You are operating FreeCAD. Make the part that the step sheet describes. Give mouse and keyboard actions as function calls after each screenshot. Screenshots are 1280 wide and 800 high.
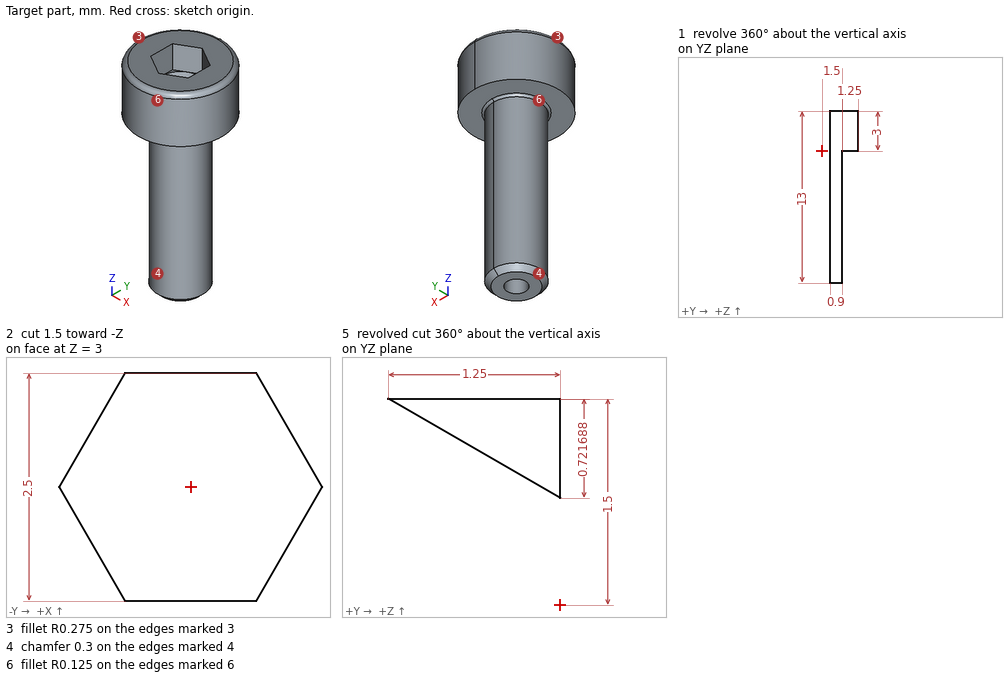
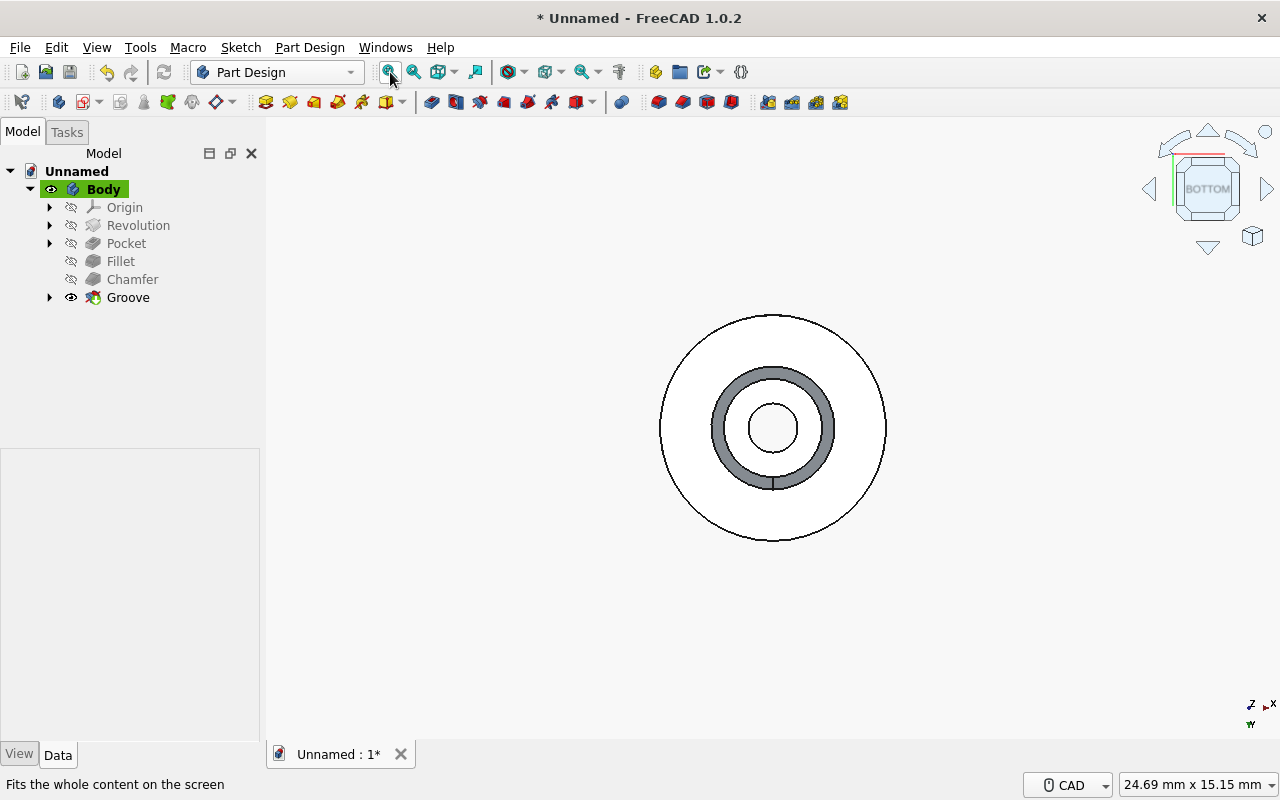
click(390, 72)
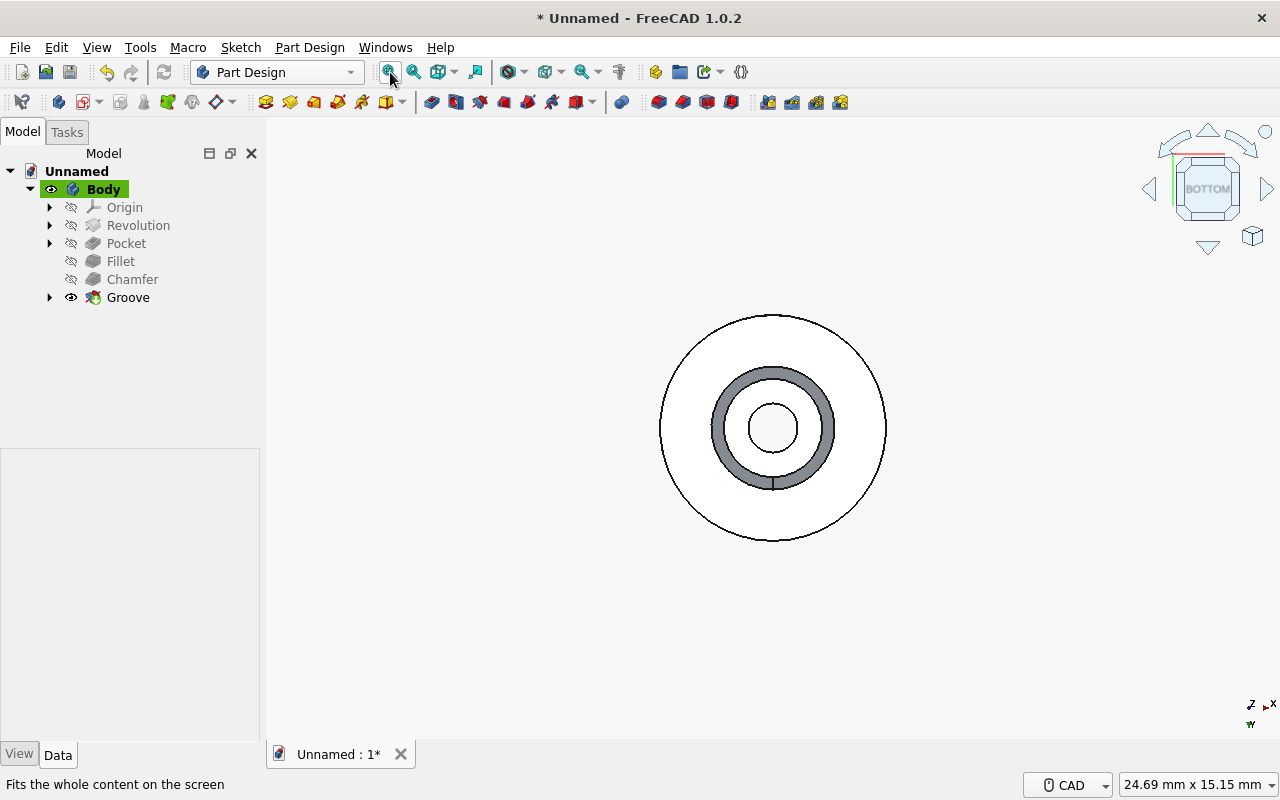
key(4)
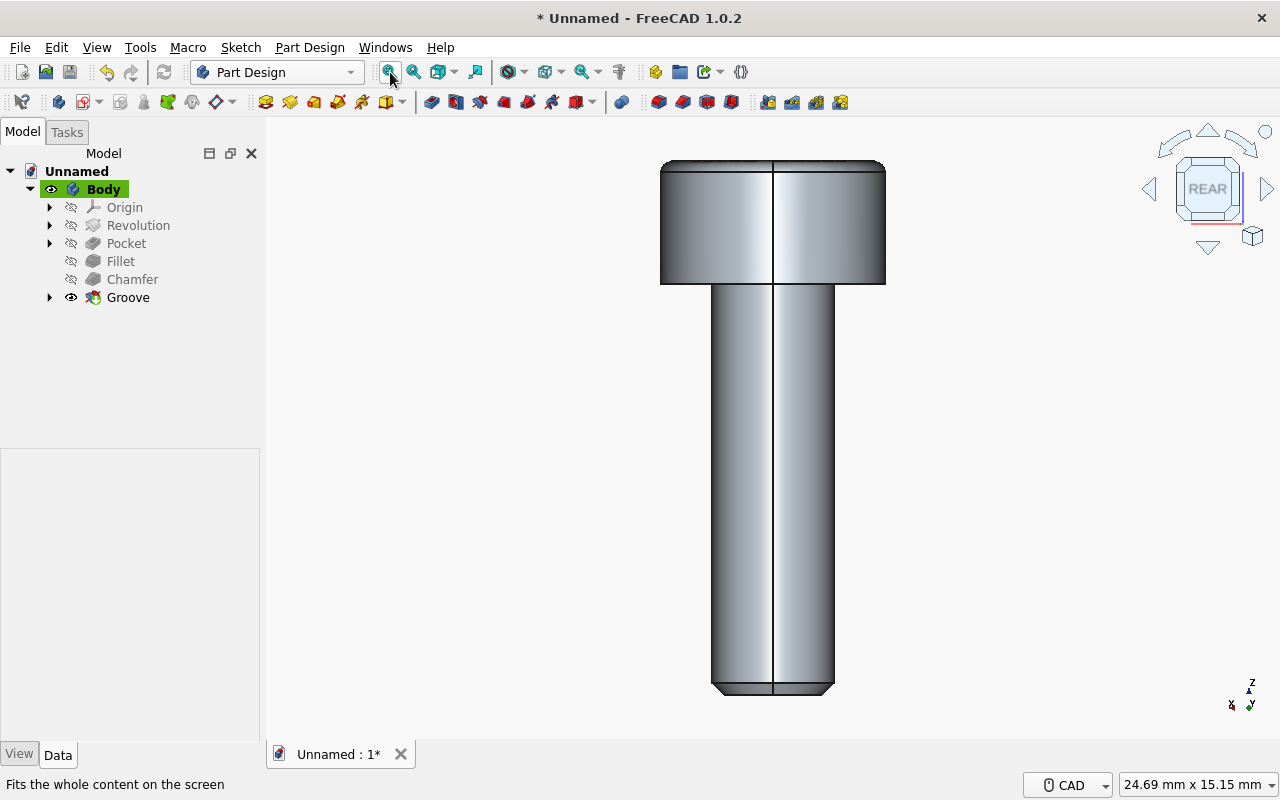
key(6)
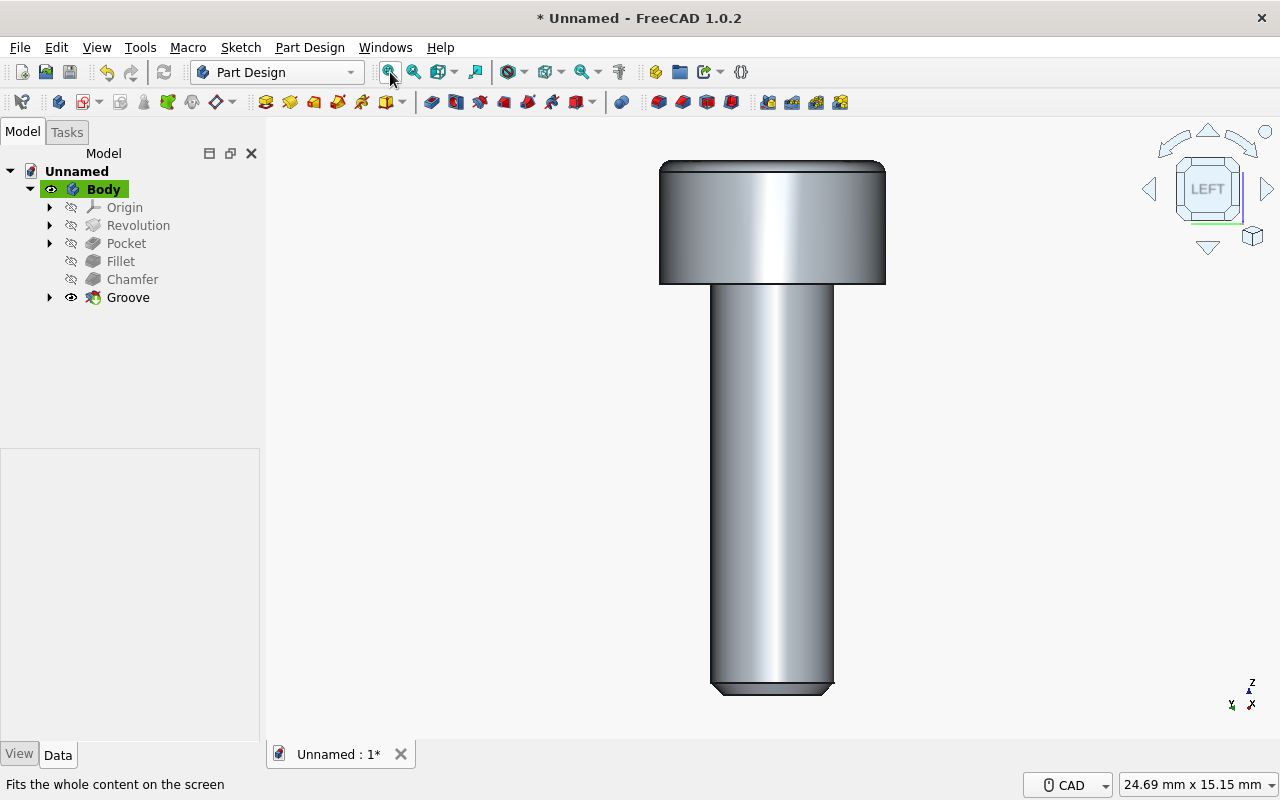
key(v)
key(3)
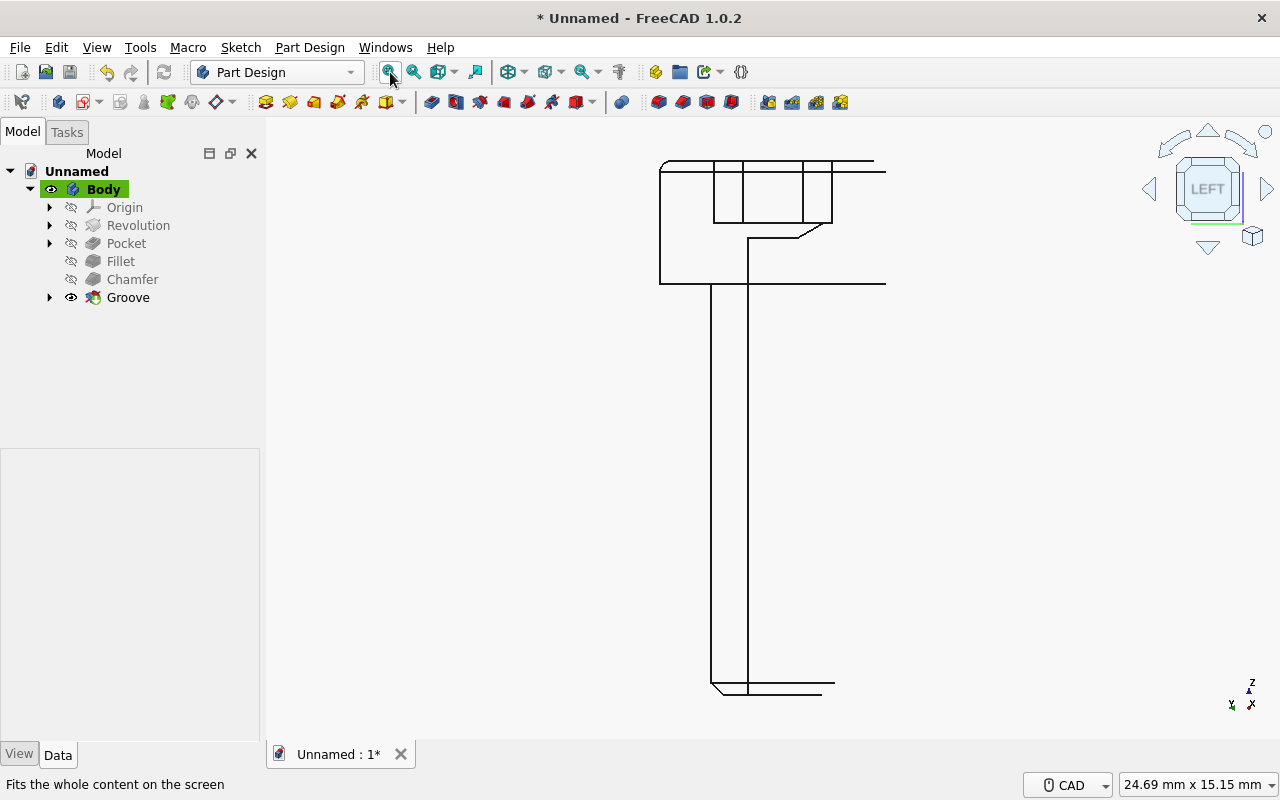
key(0)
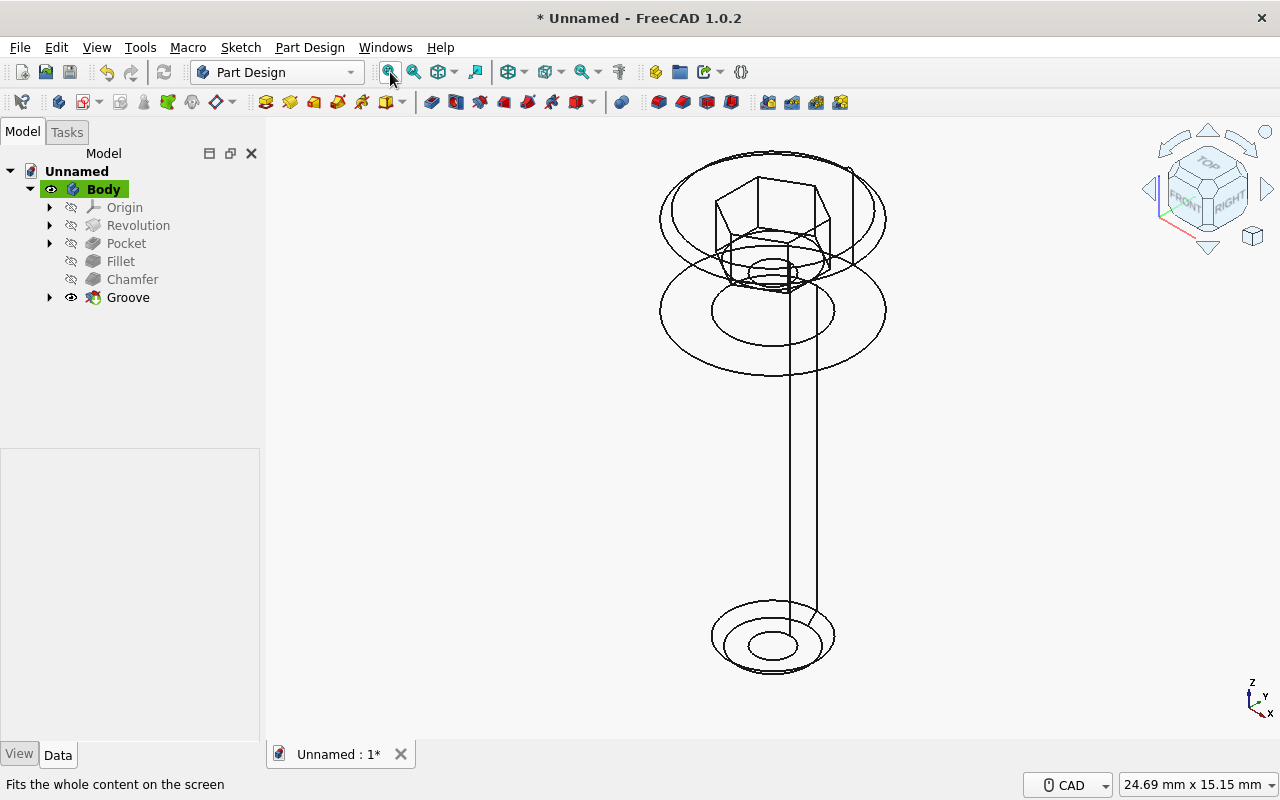
click(729, 335)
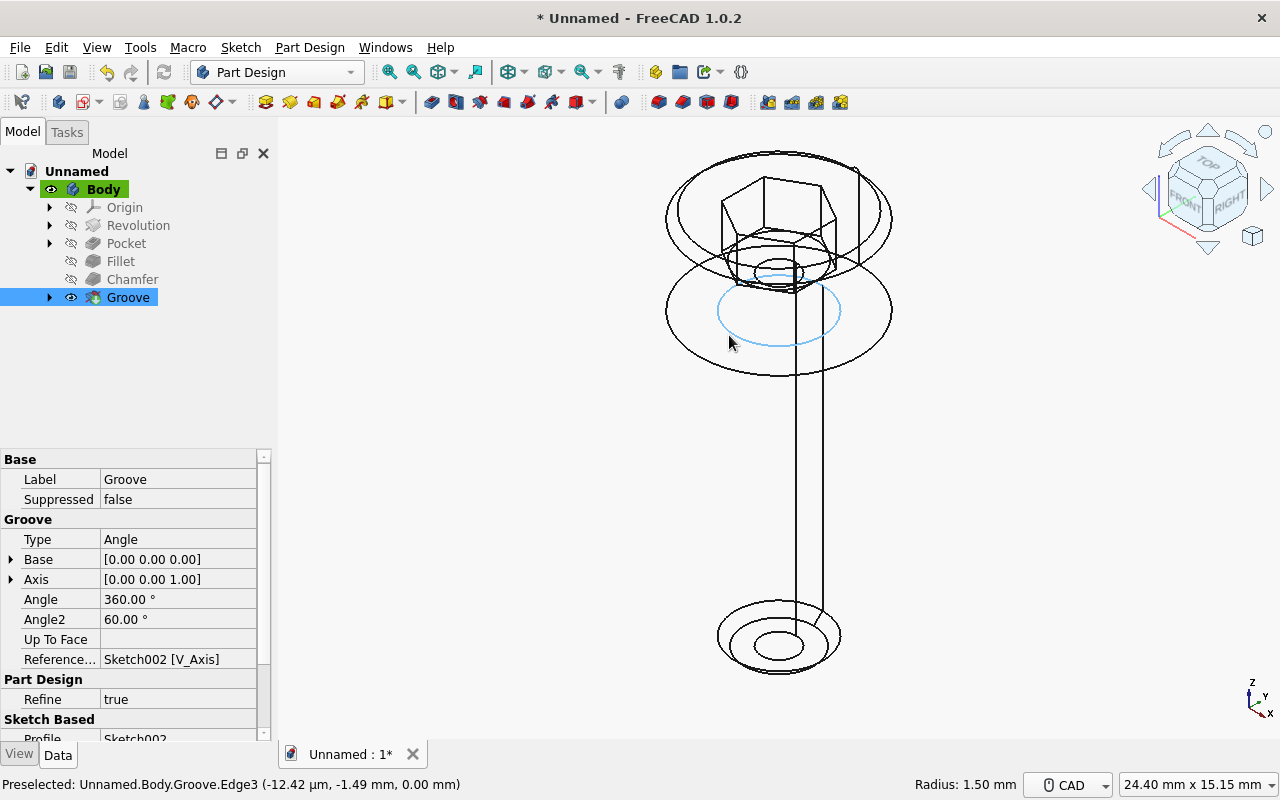
key(v)
key(1)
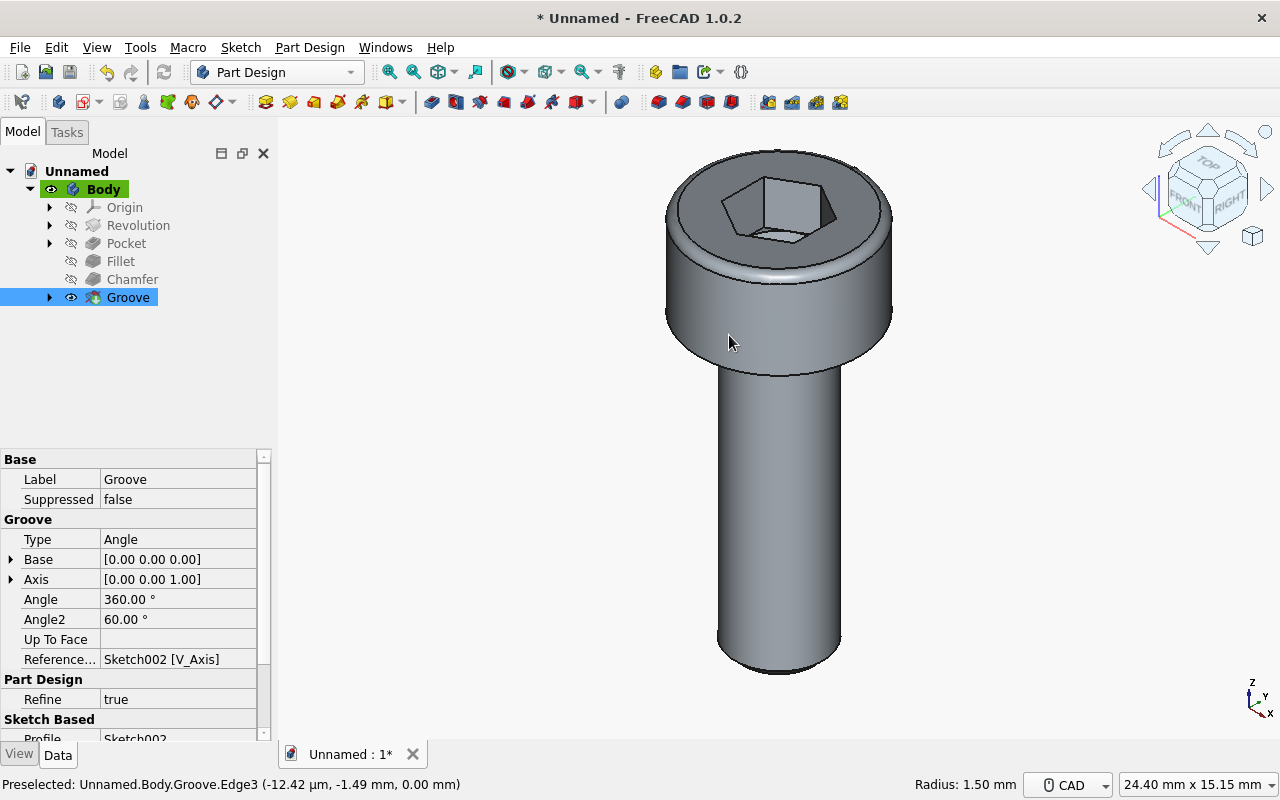
click(660, 102)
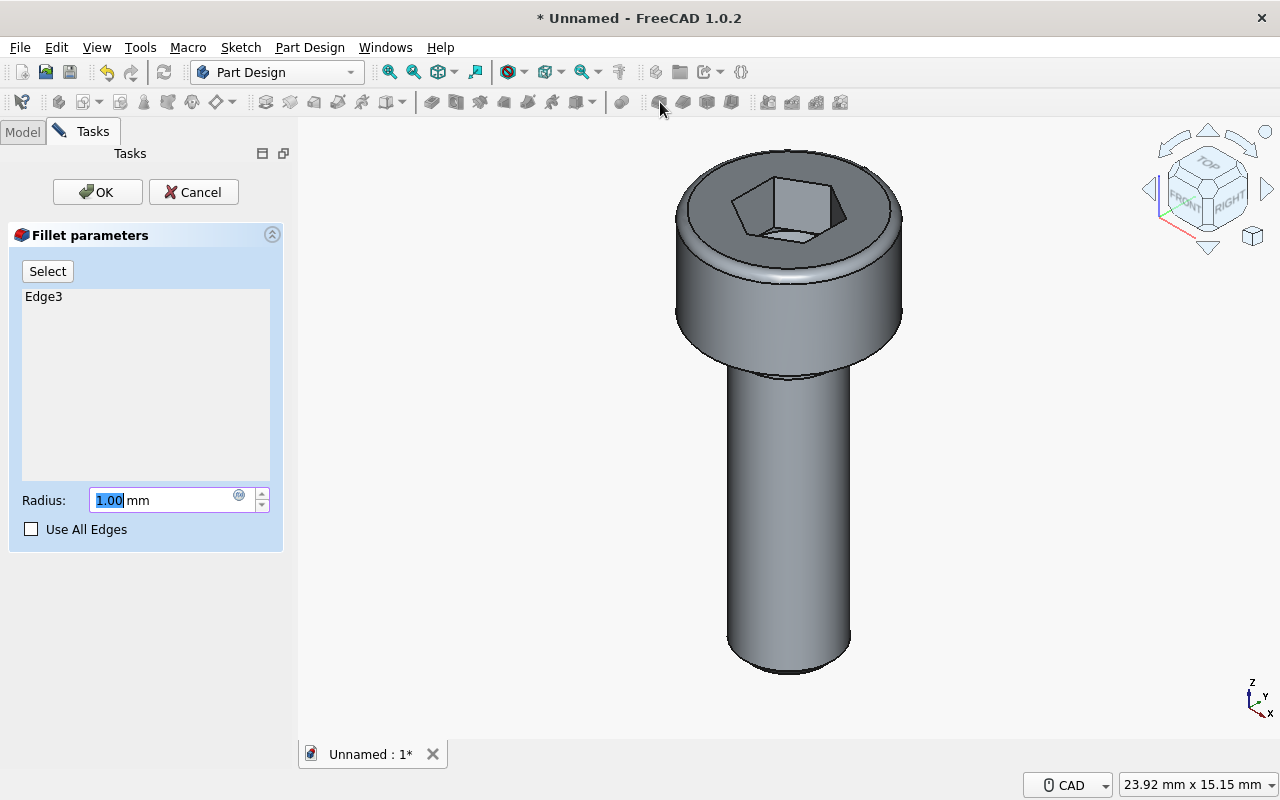
text(0.125)
key(Tab)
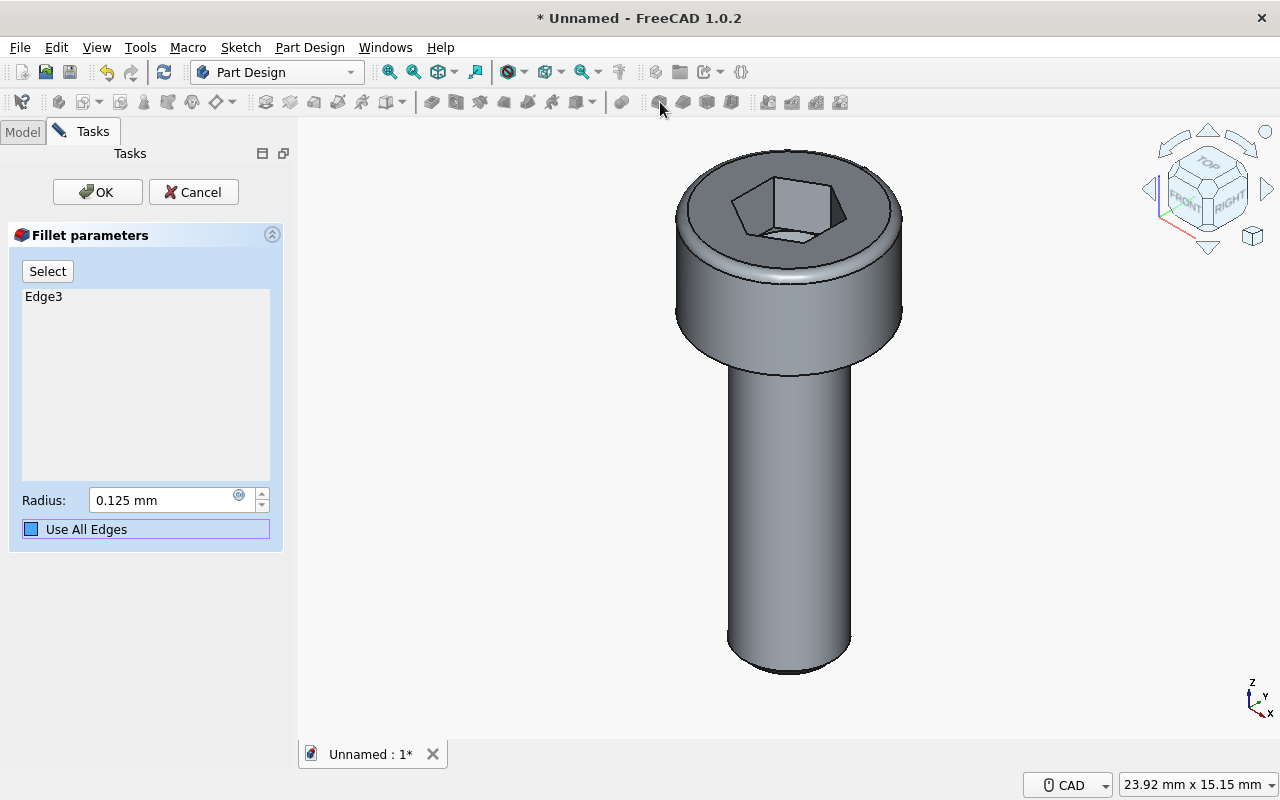
click(98, 192)